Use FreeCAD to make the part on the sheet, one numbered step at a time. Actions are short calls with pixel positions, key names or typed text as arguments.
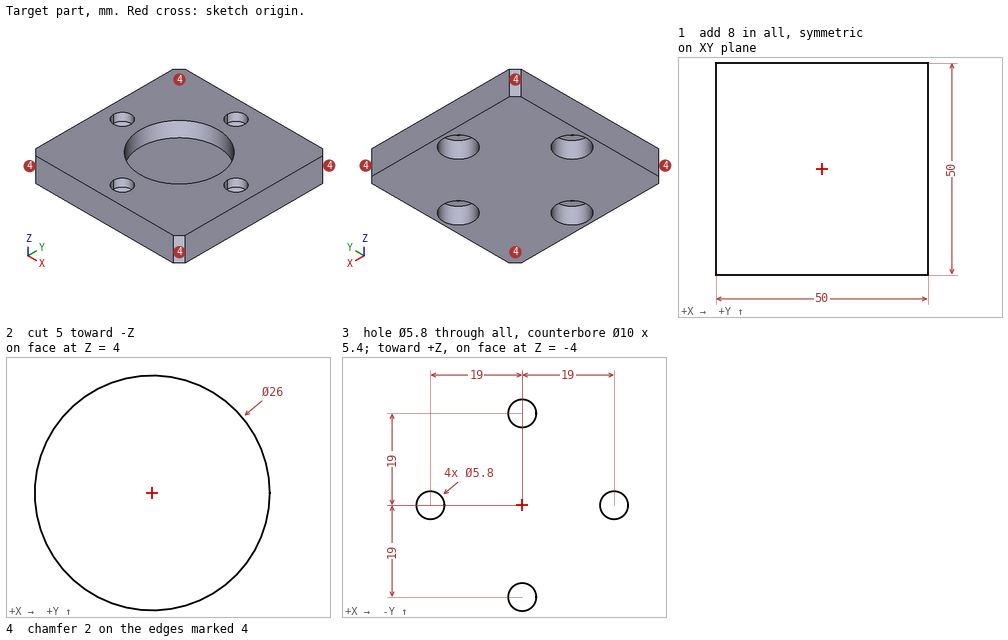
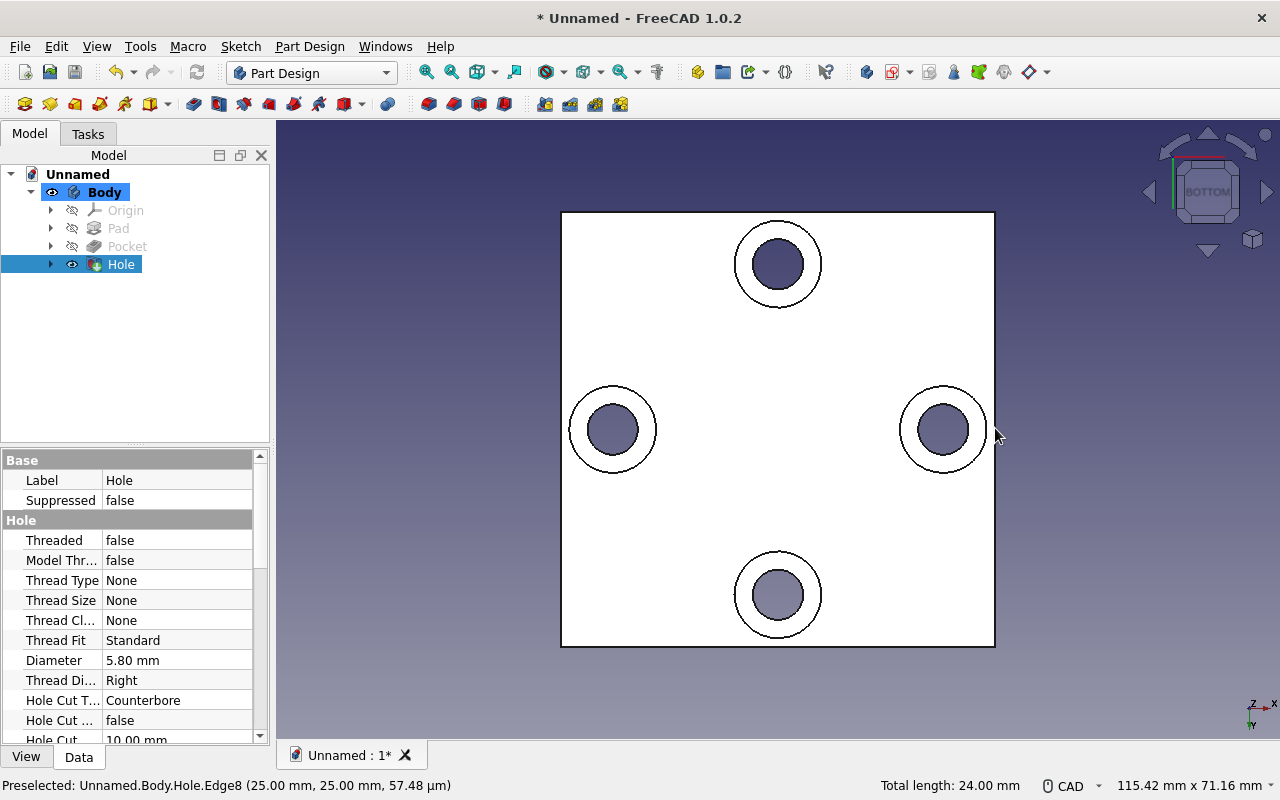
key(4)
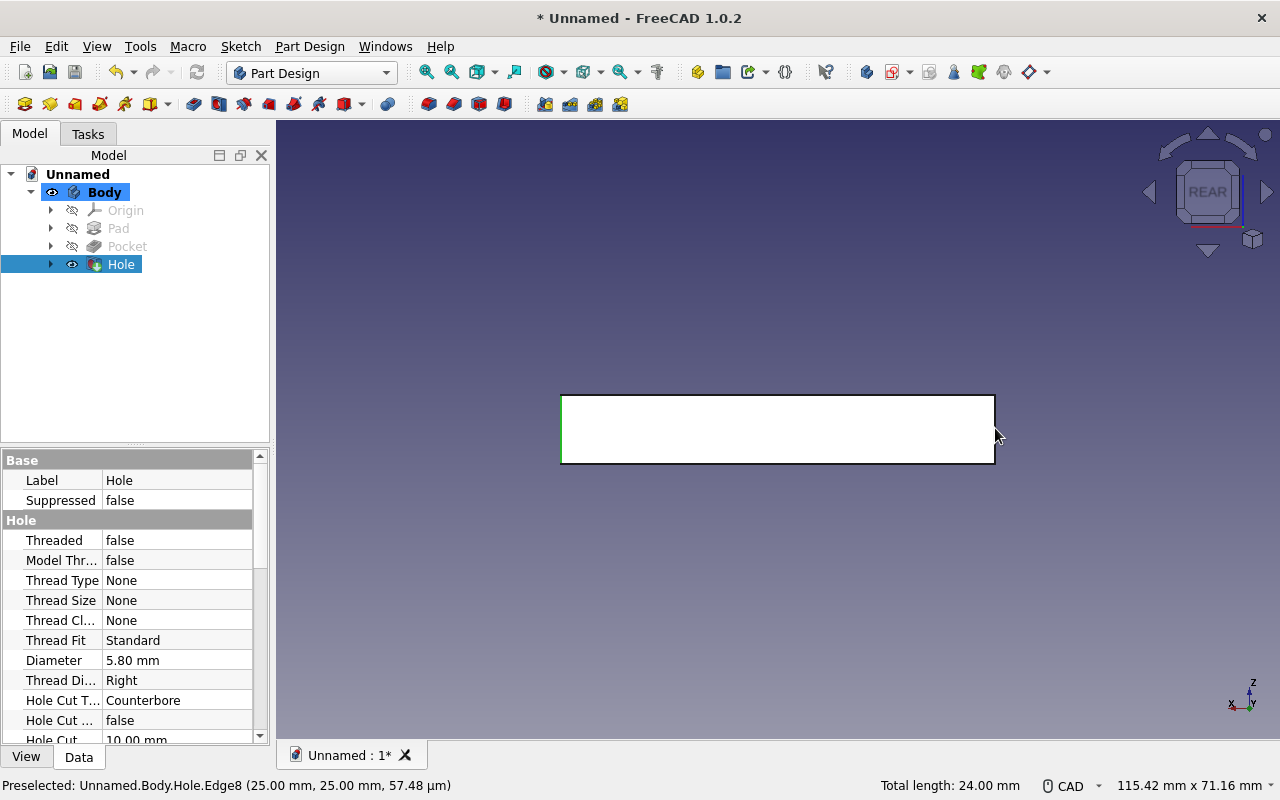
click(427, 72)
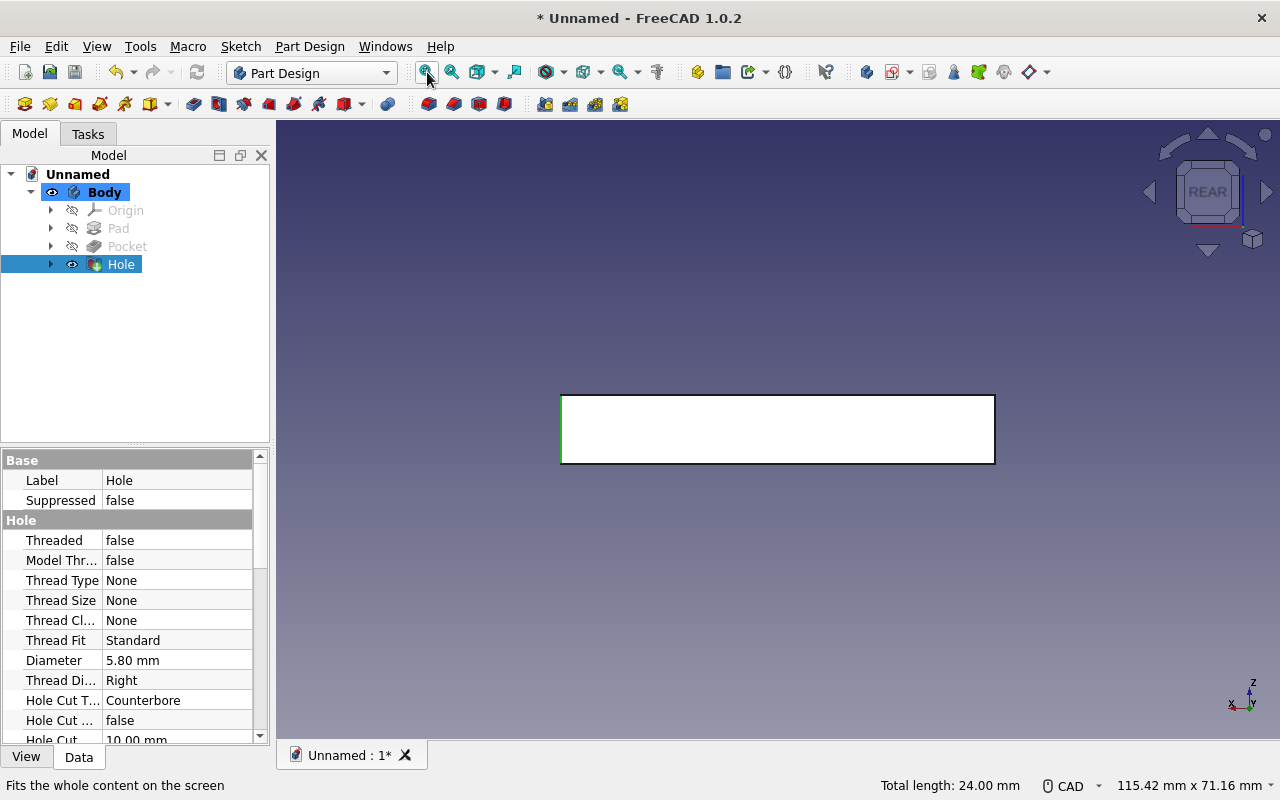
click(995, 429, ctrl)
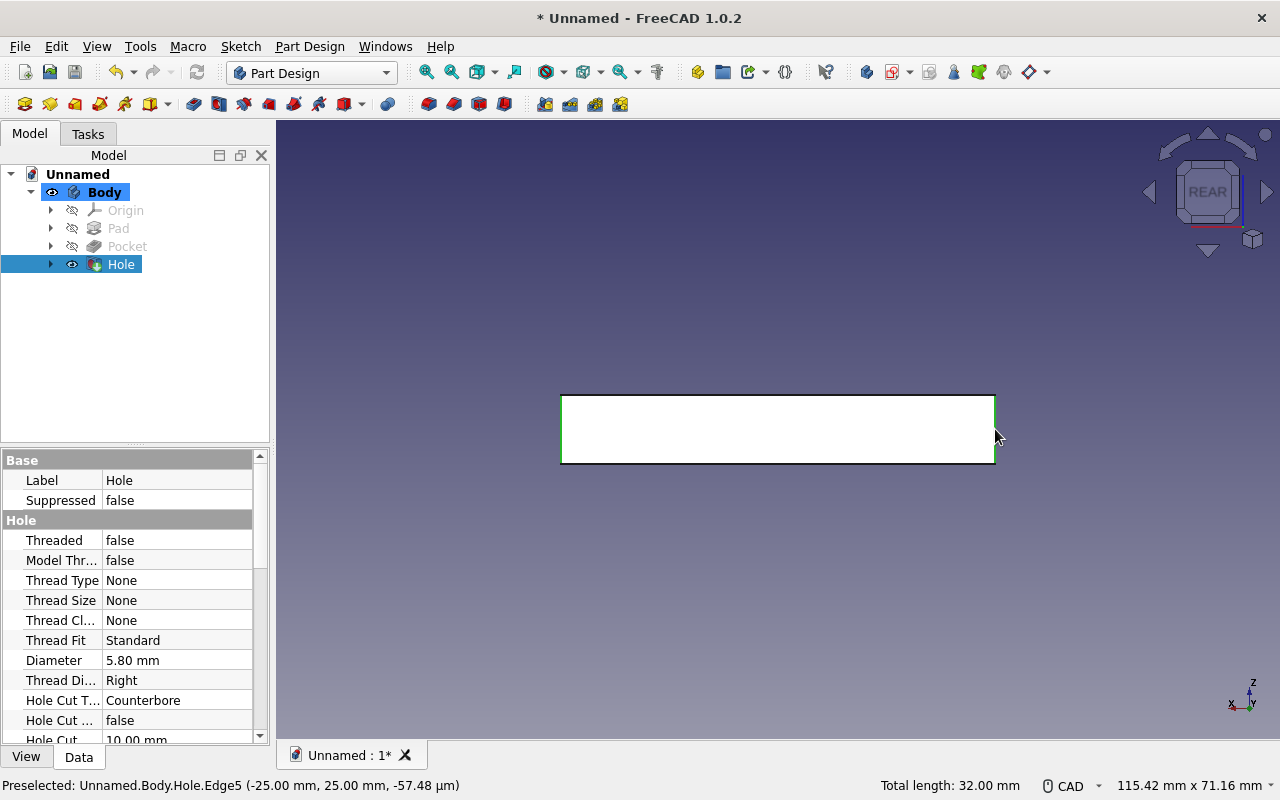
click(454, 104)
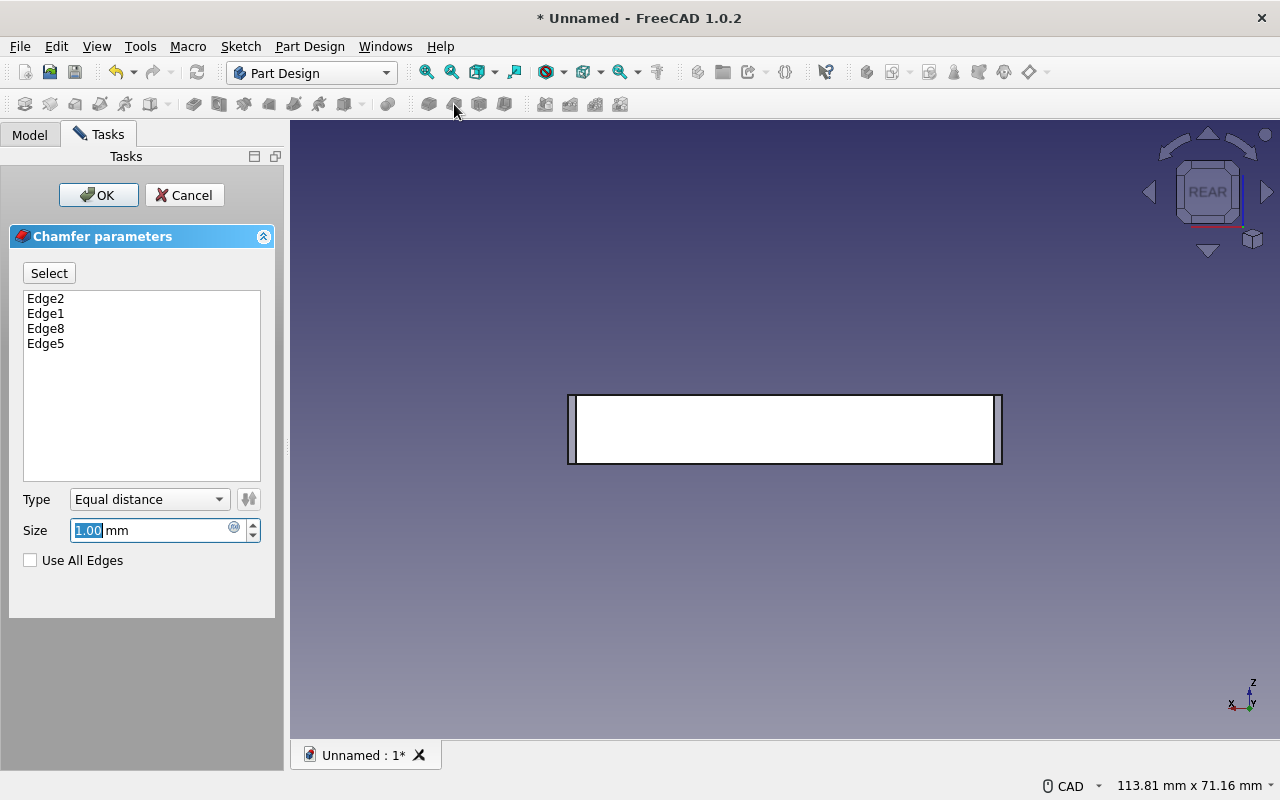
text(2)
key(Tab)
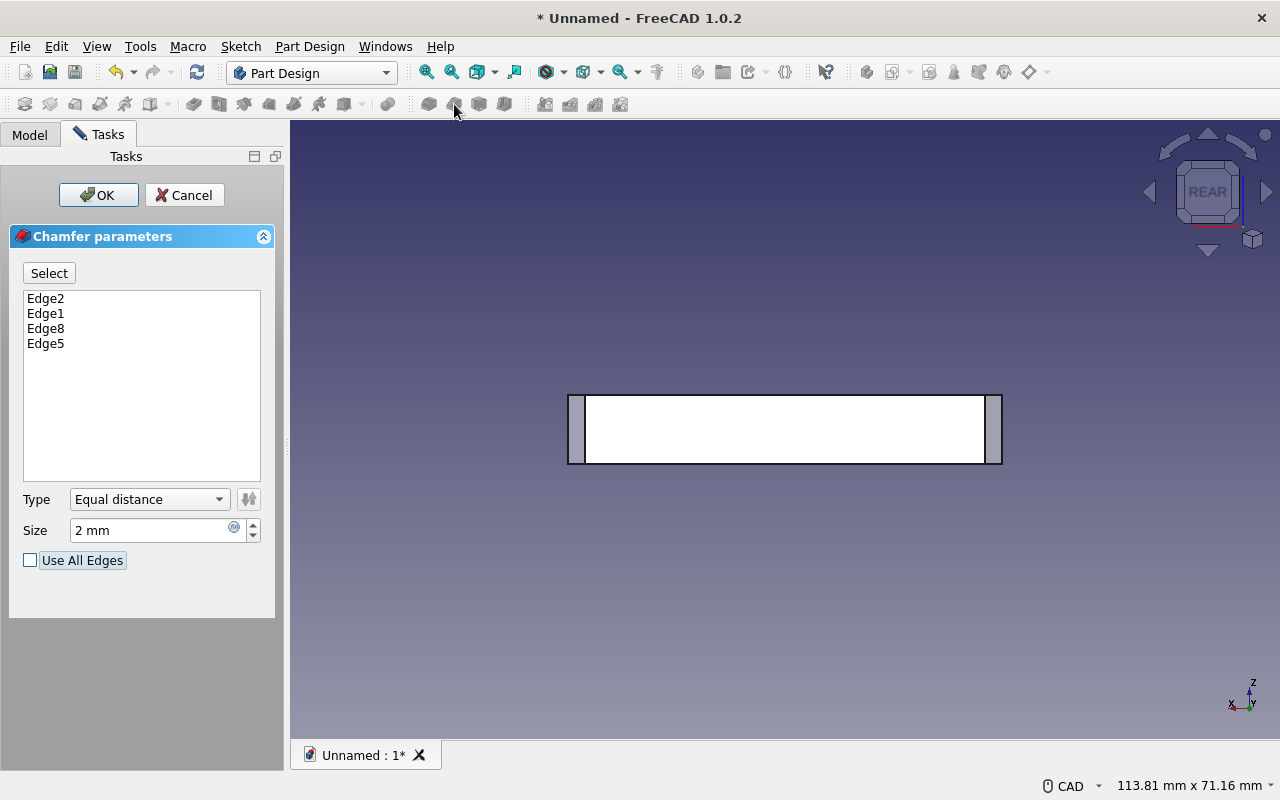
click(99, 195)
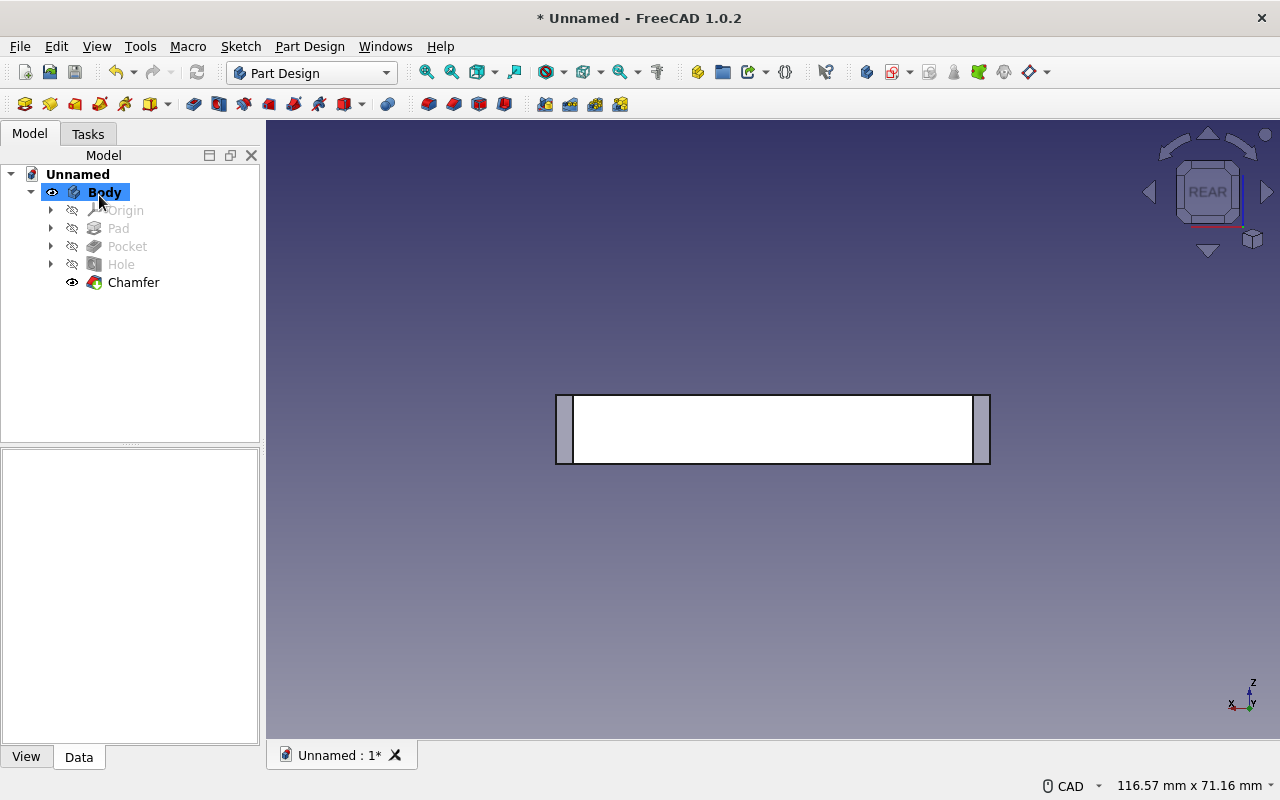
key(0)